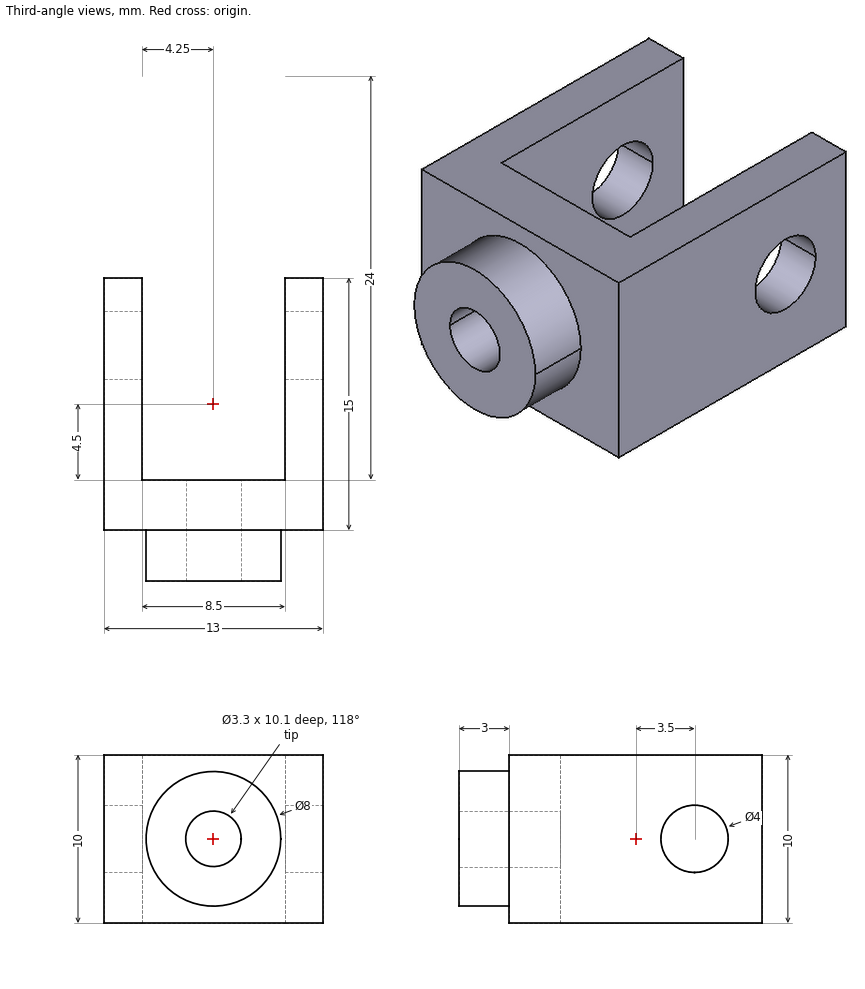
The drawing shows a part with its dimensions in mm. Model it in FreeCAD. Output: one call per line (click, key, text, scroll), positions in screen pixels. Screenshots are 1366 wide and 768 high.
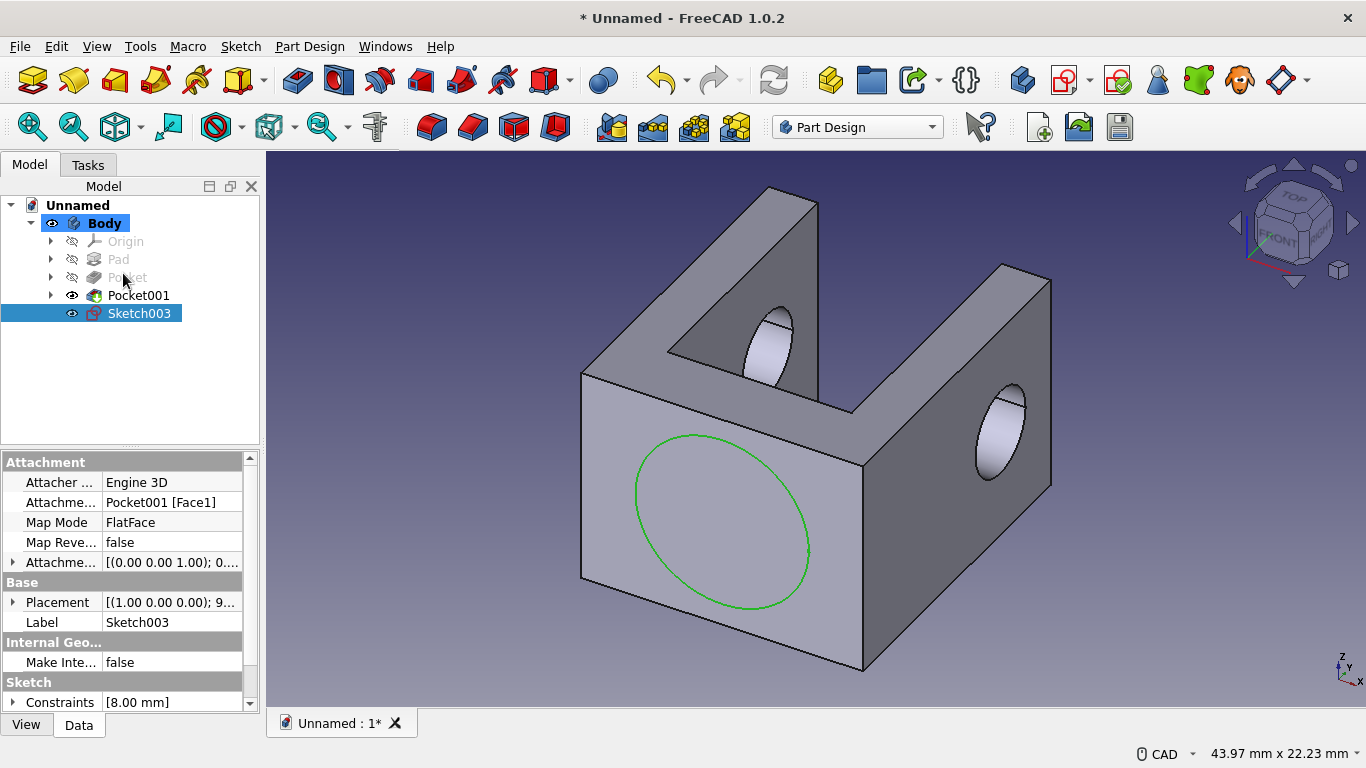
click(33, 80)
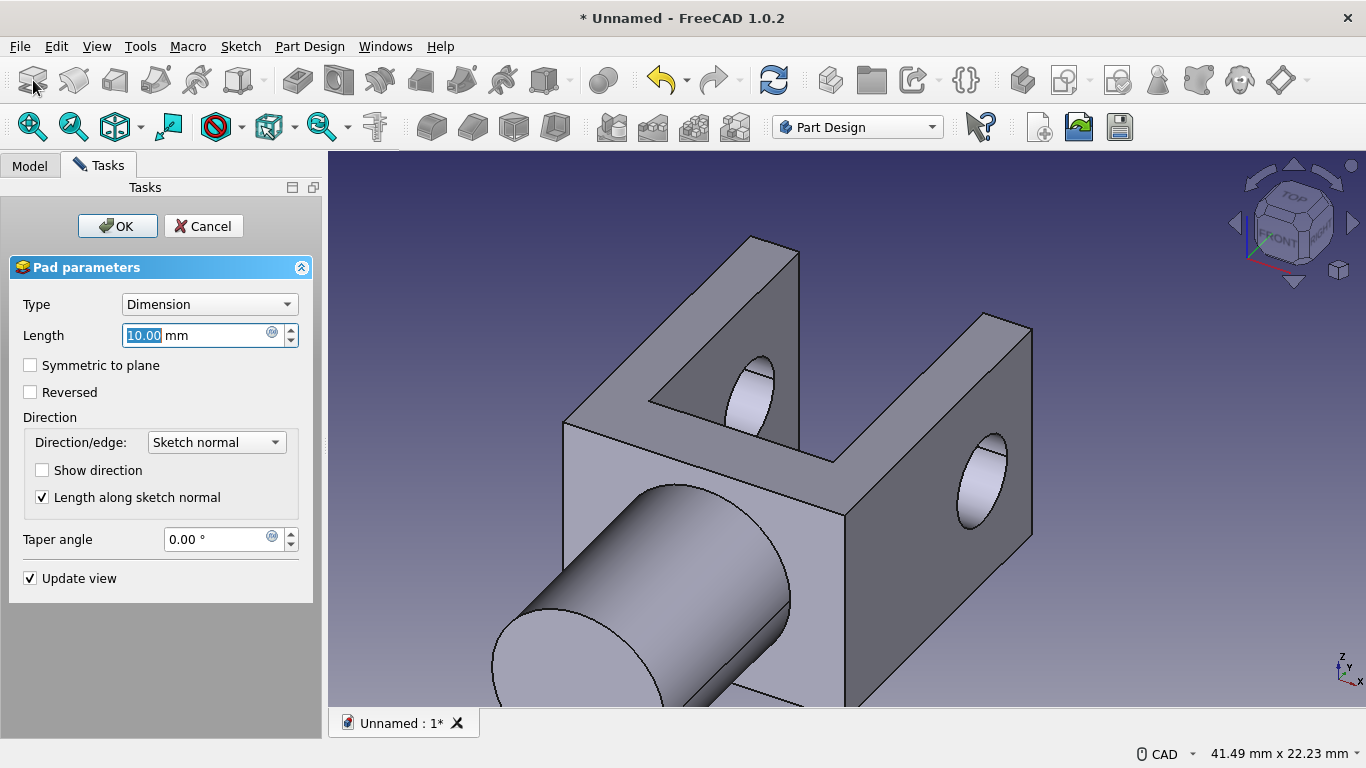
text(3)
key(Tab)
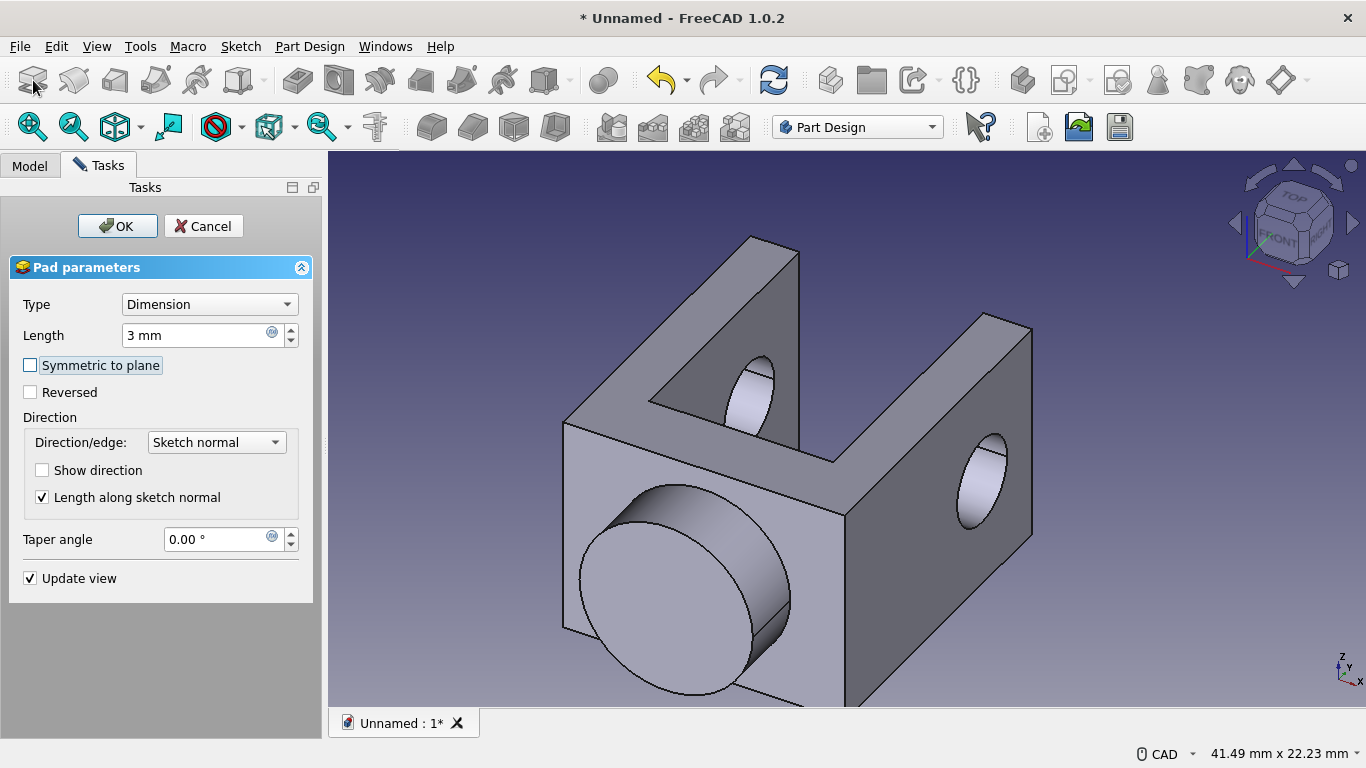
click(118, 226)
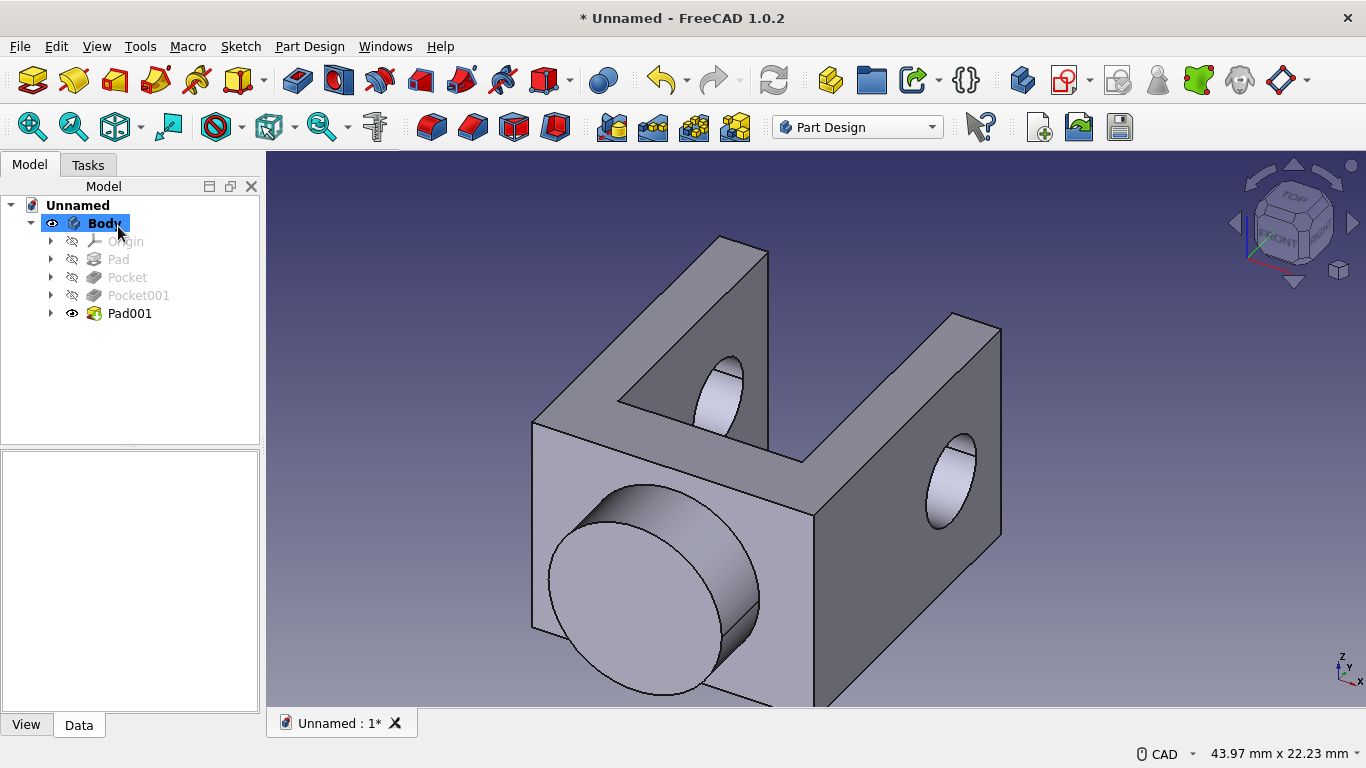
click(33, 128)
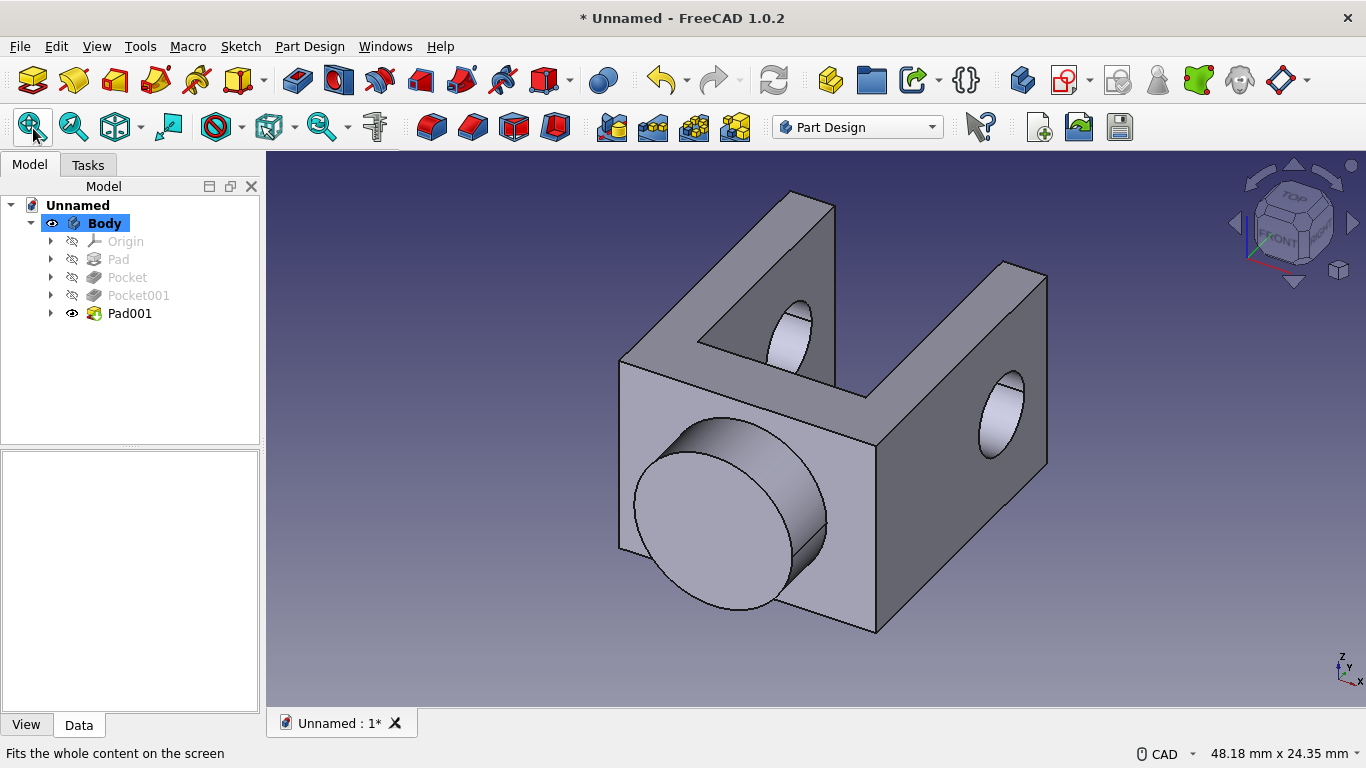
click(713, 530)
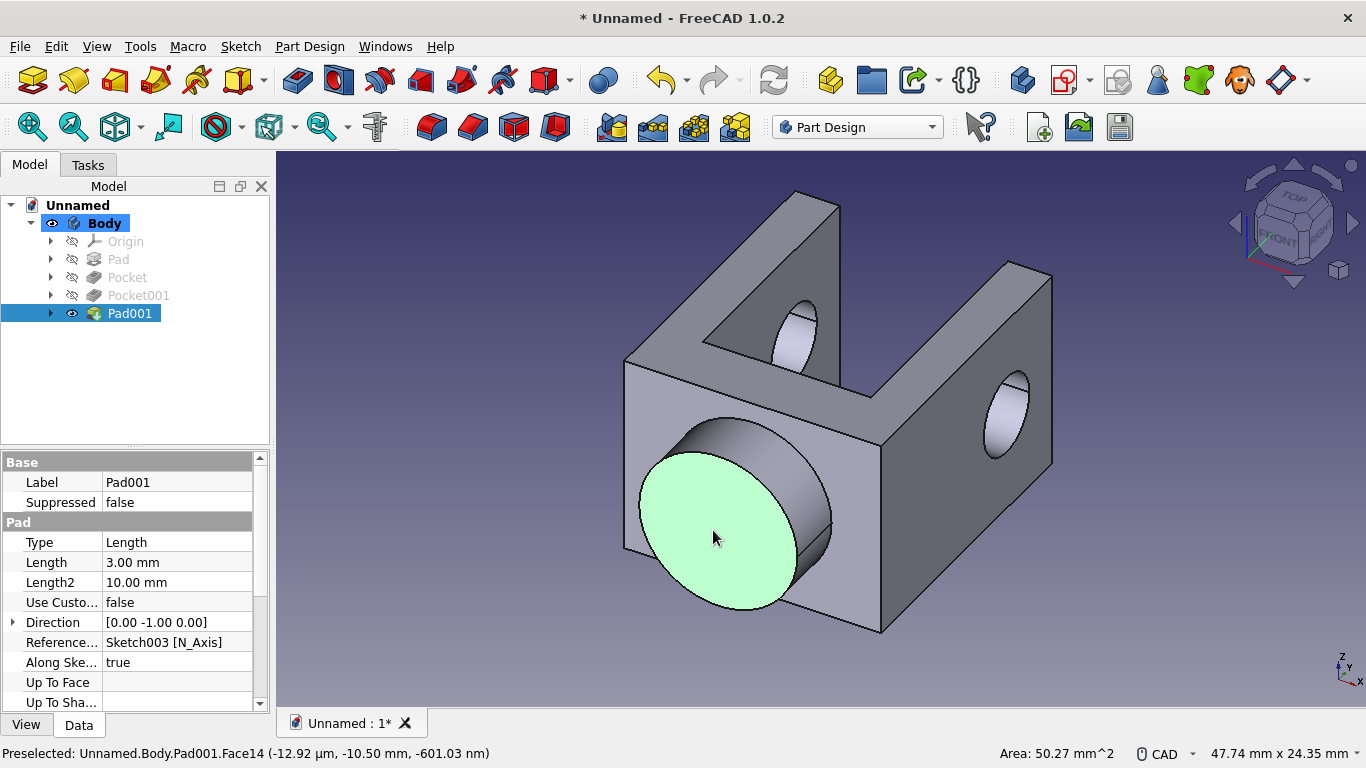
click(1064, 80)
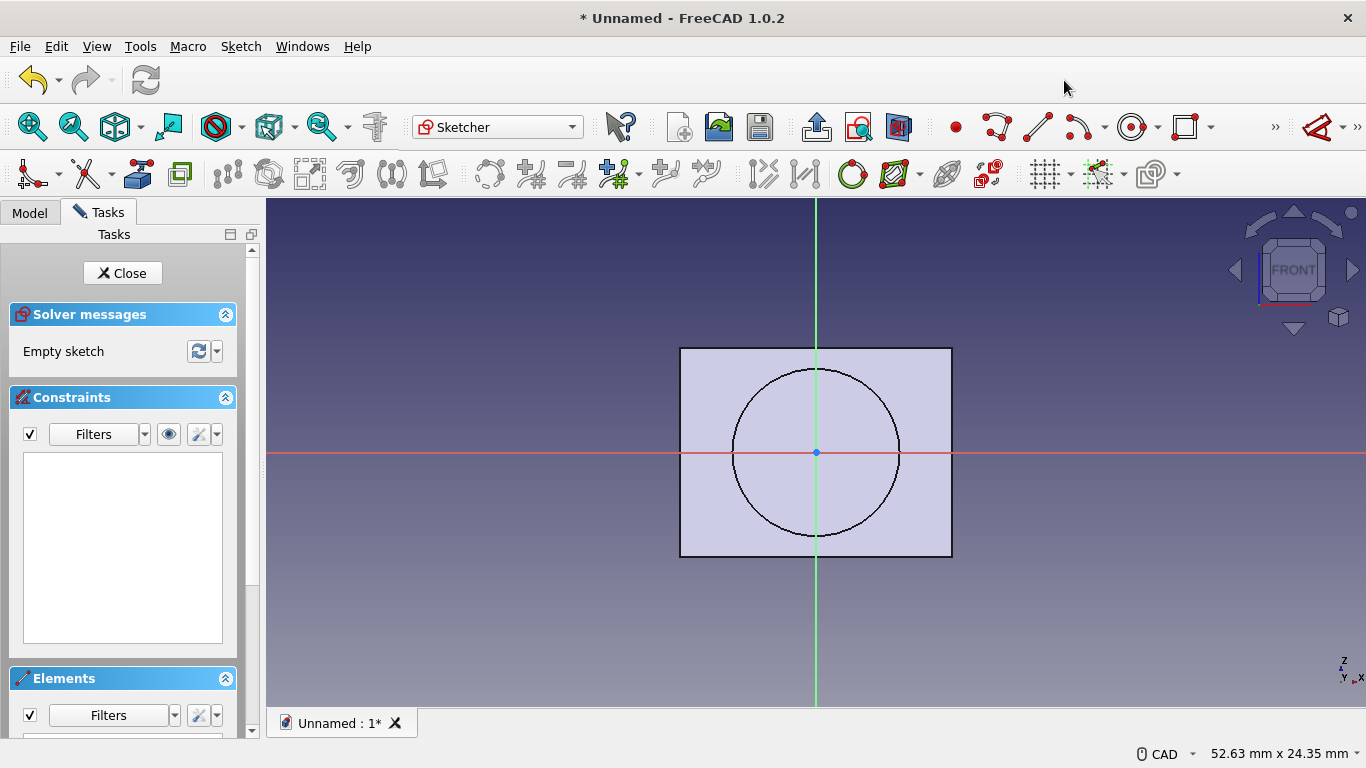
scroll(833, 452, up, 8)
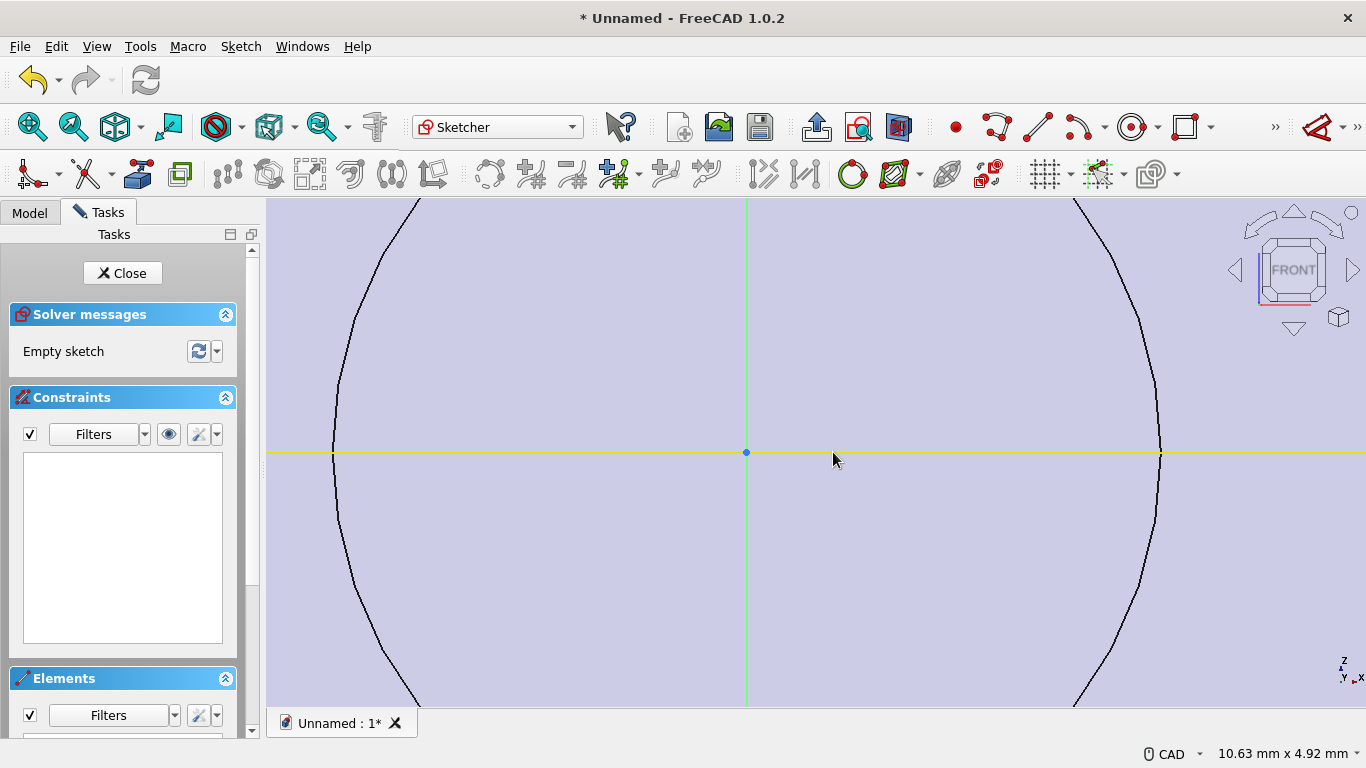
key(g)
key(c)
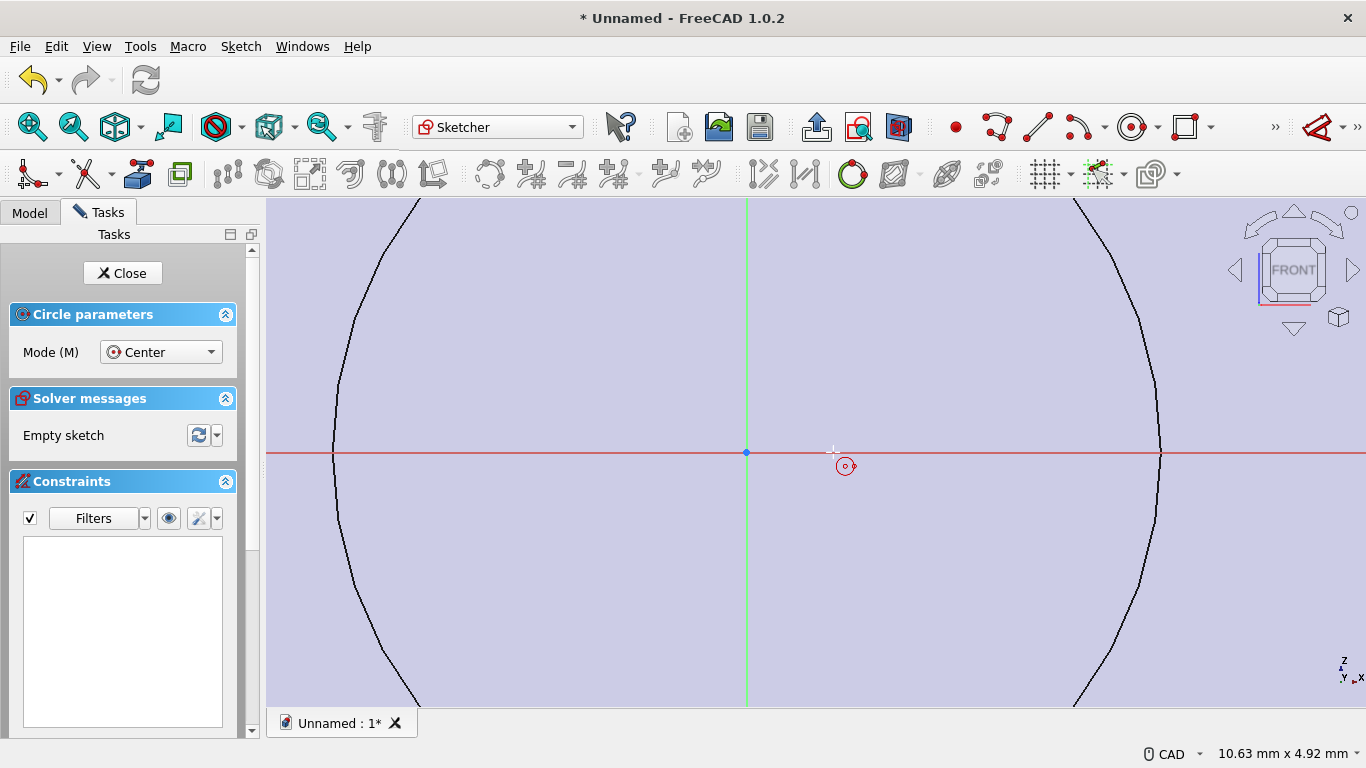
click(747, 452)
move(868, 332)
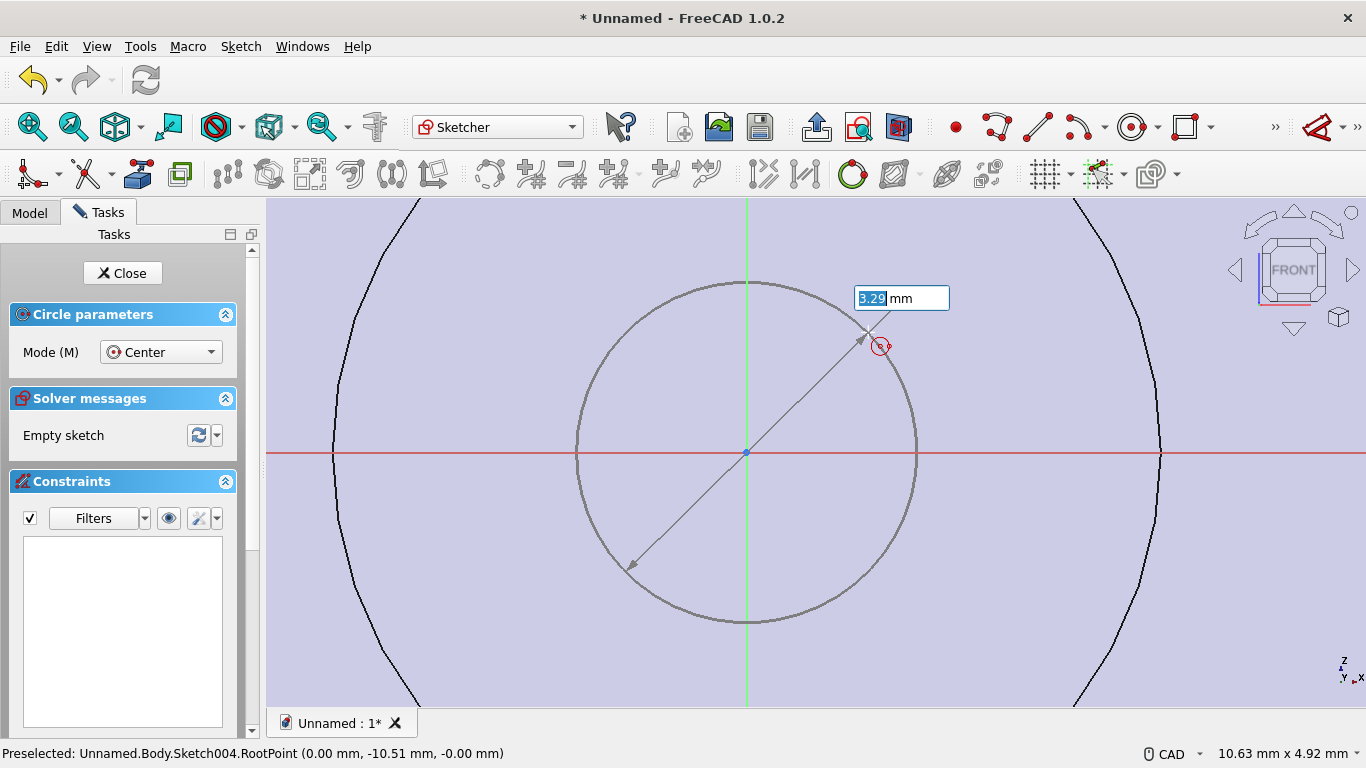
text(3.3)
key(Return)
key(Escape)